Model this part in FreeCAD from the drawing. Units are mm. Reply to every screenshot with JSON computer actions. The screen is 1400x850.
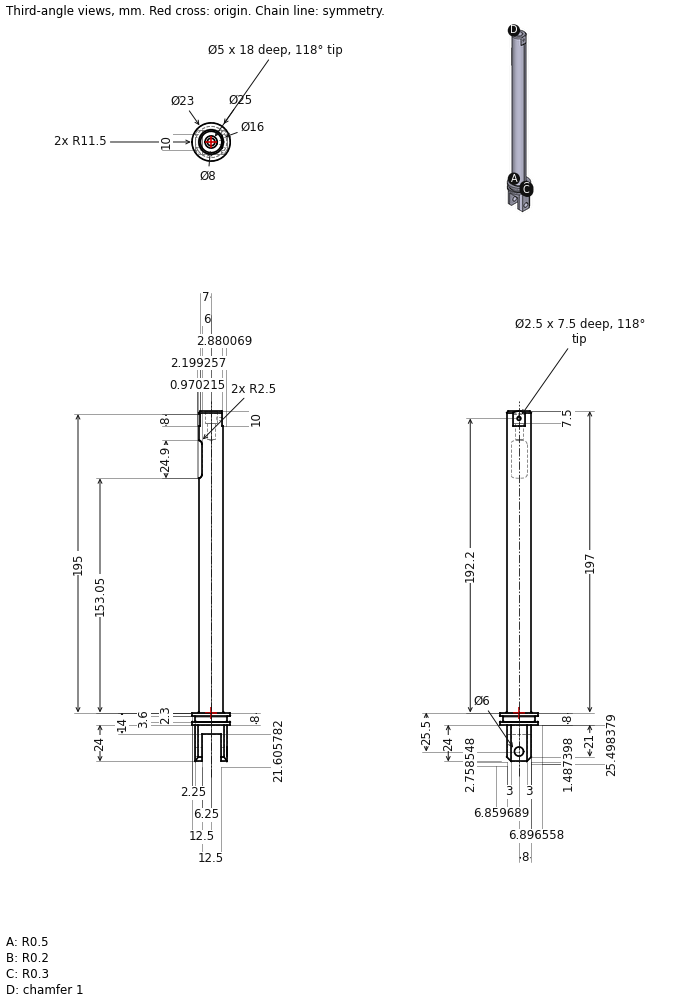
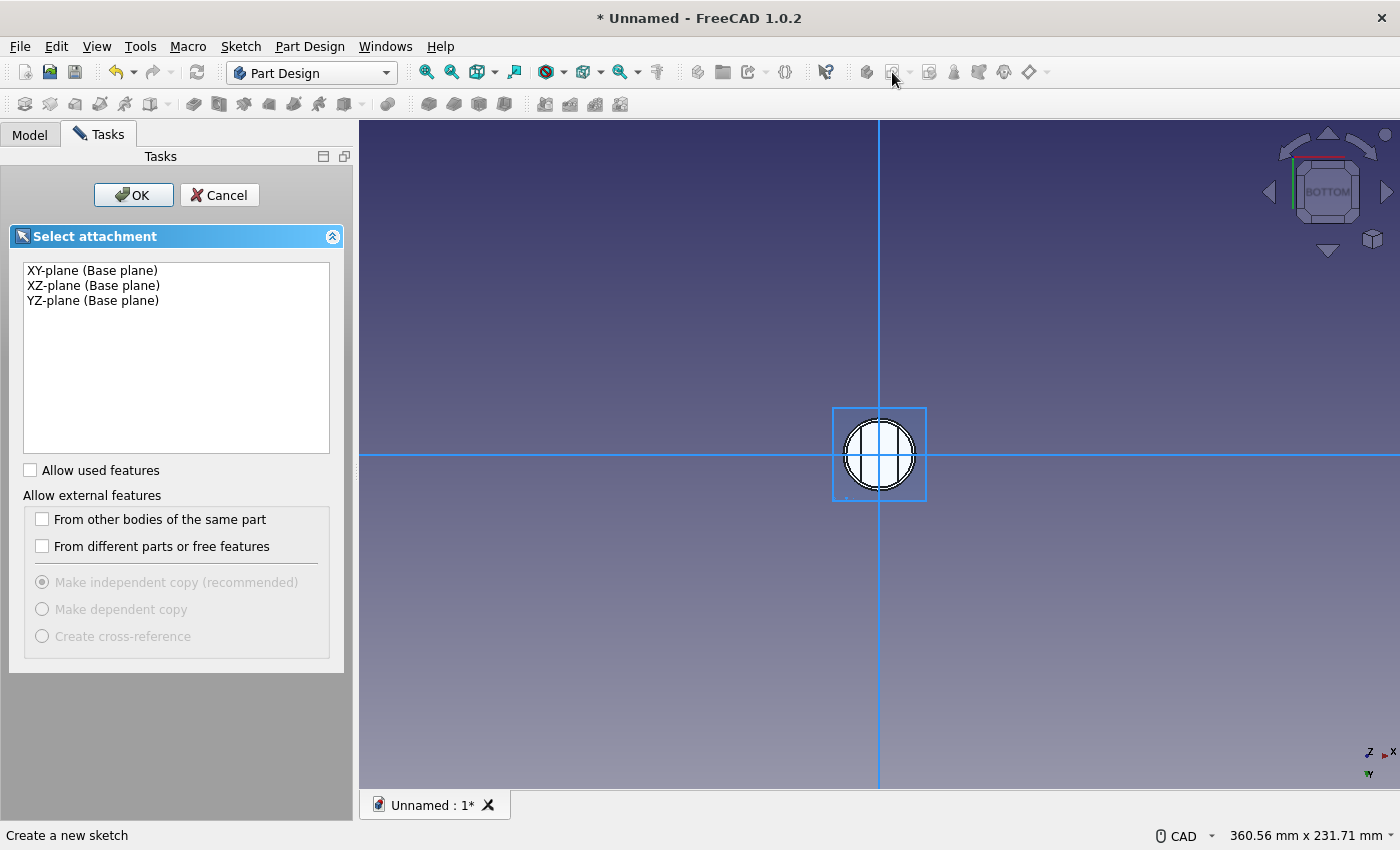
{"action": "left_click", "coordinate": [84, 300]}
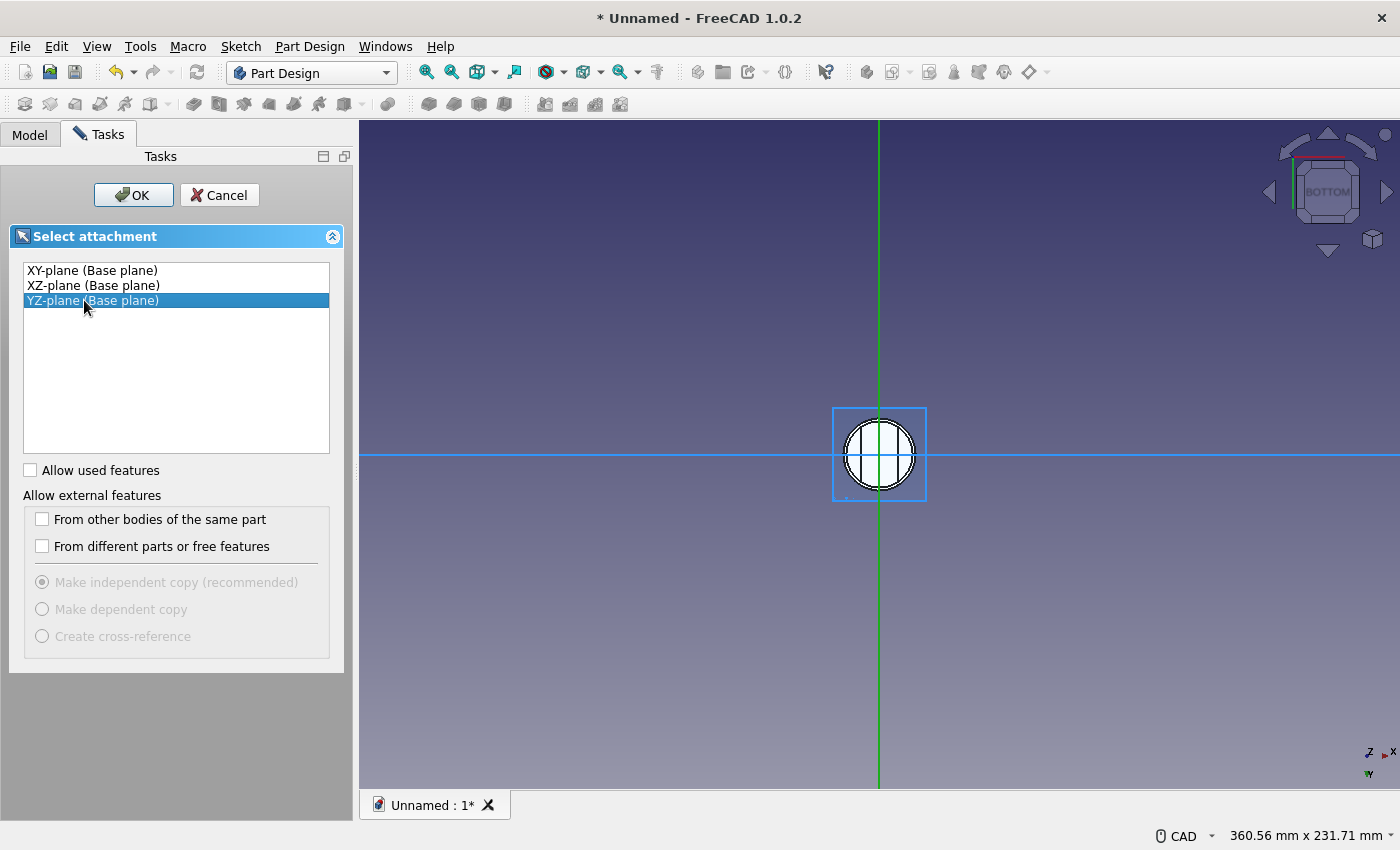
{"action": "left_click", "coordinate": [134, 195]}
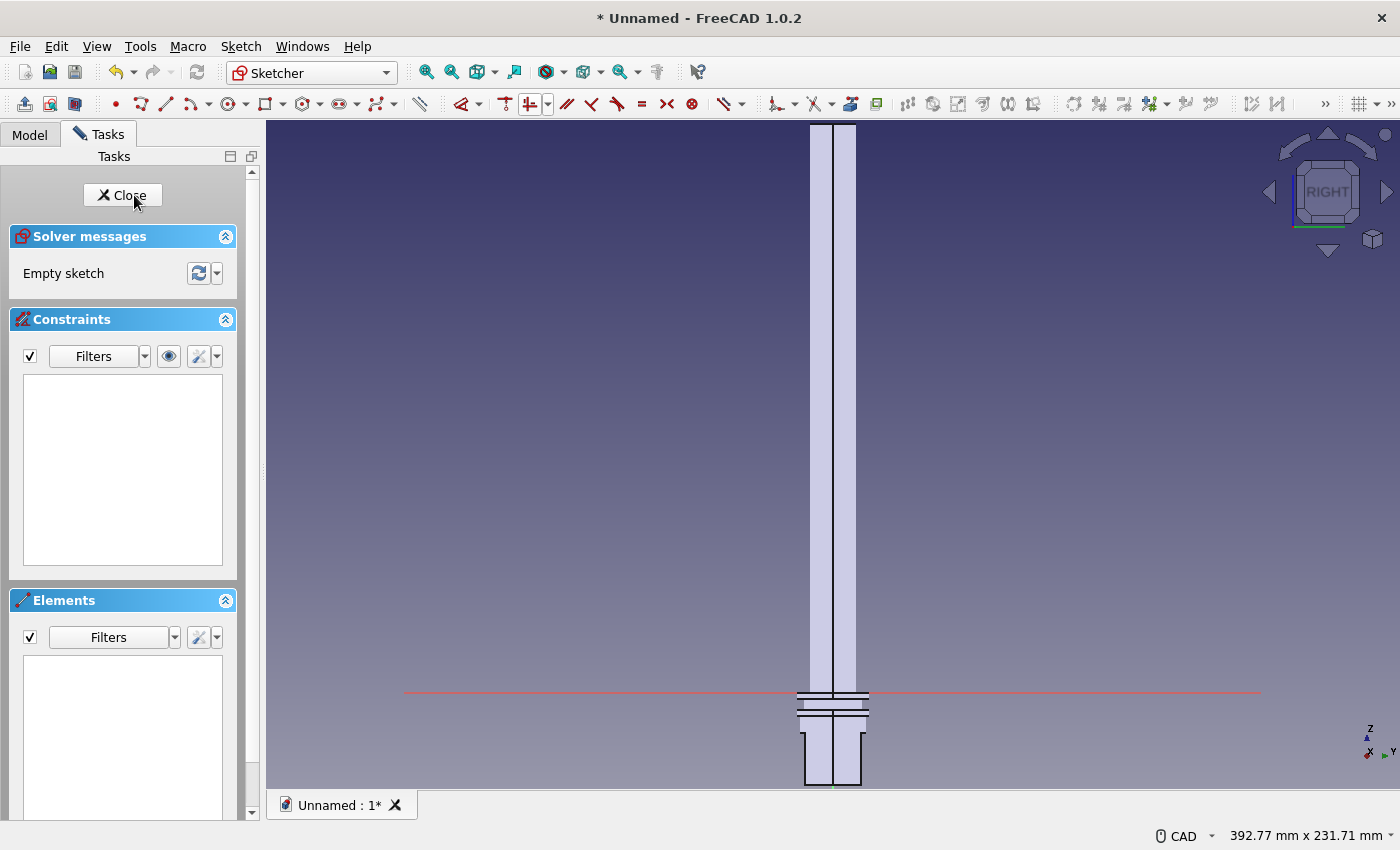
{"action": "left_click", "coordinate": [75, 104]}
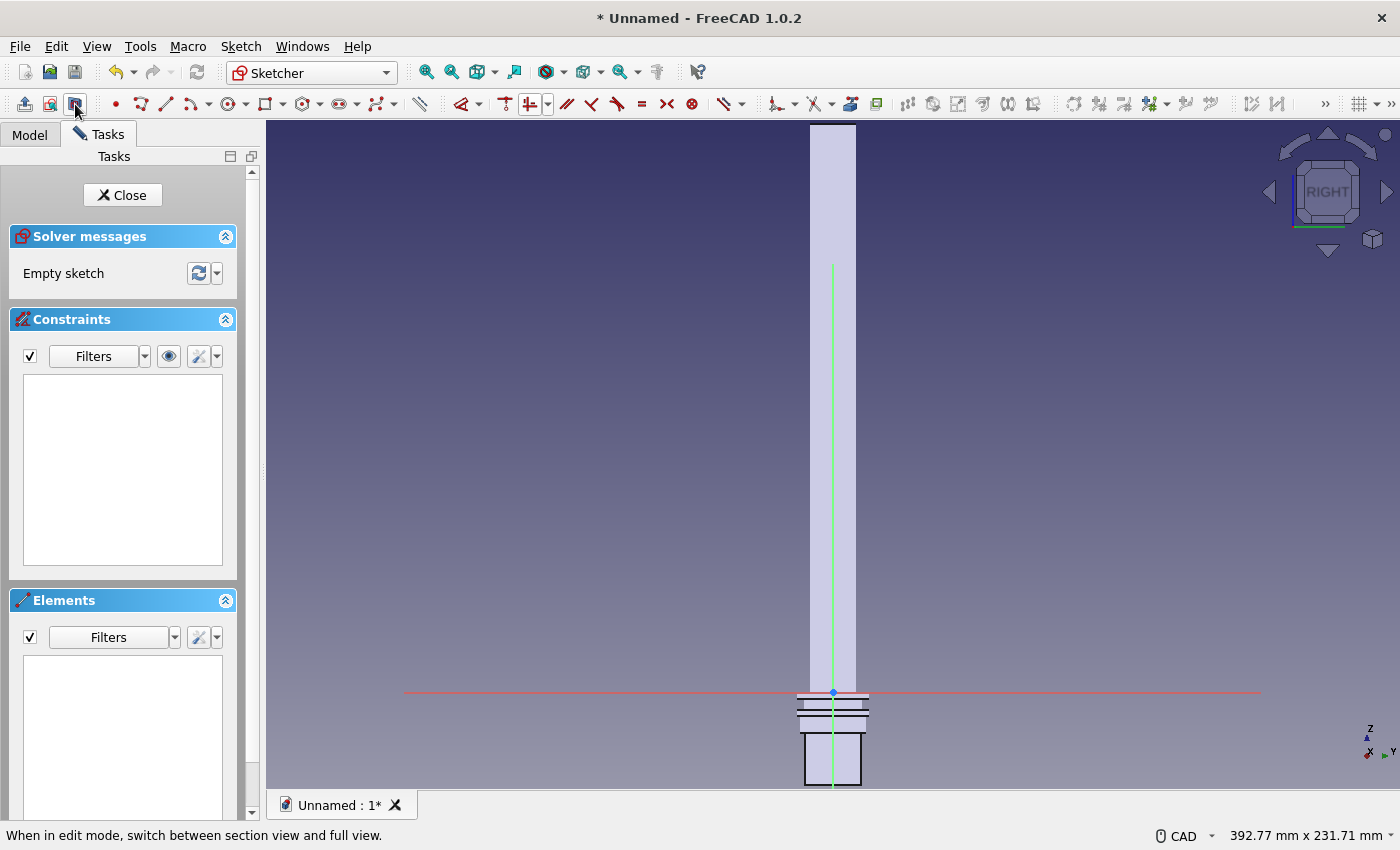
{"action": "scroll", "coordinate": [764, 454], "scroll_direction": "down", "scroll_amount": 5}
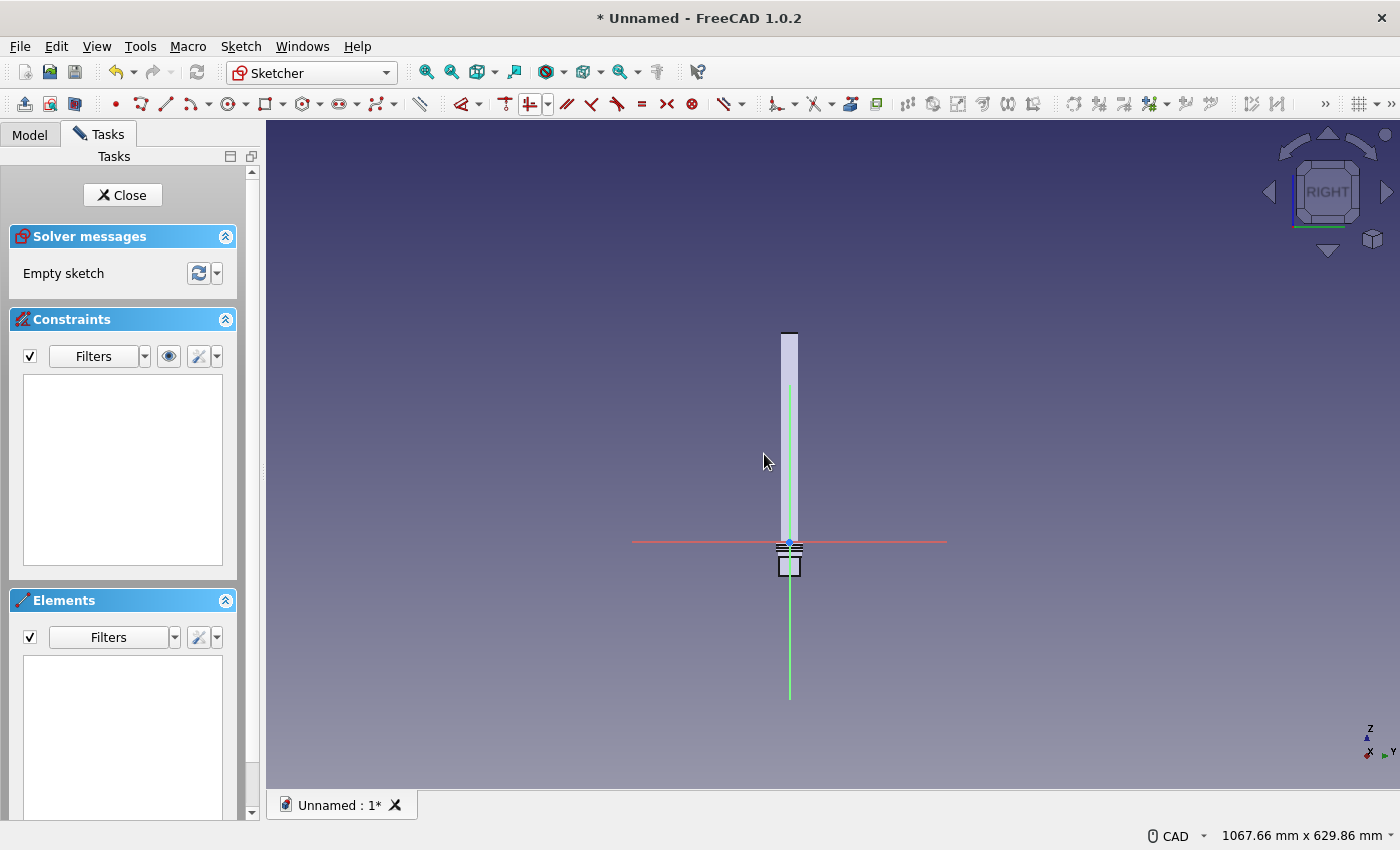
{"action": "scroll", "coordinate": [792, 571], "scroll_direction": "up", "scroll_amount": 12}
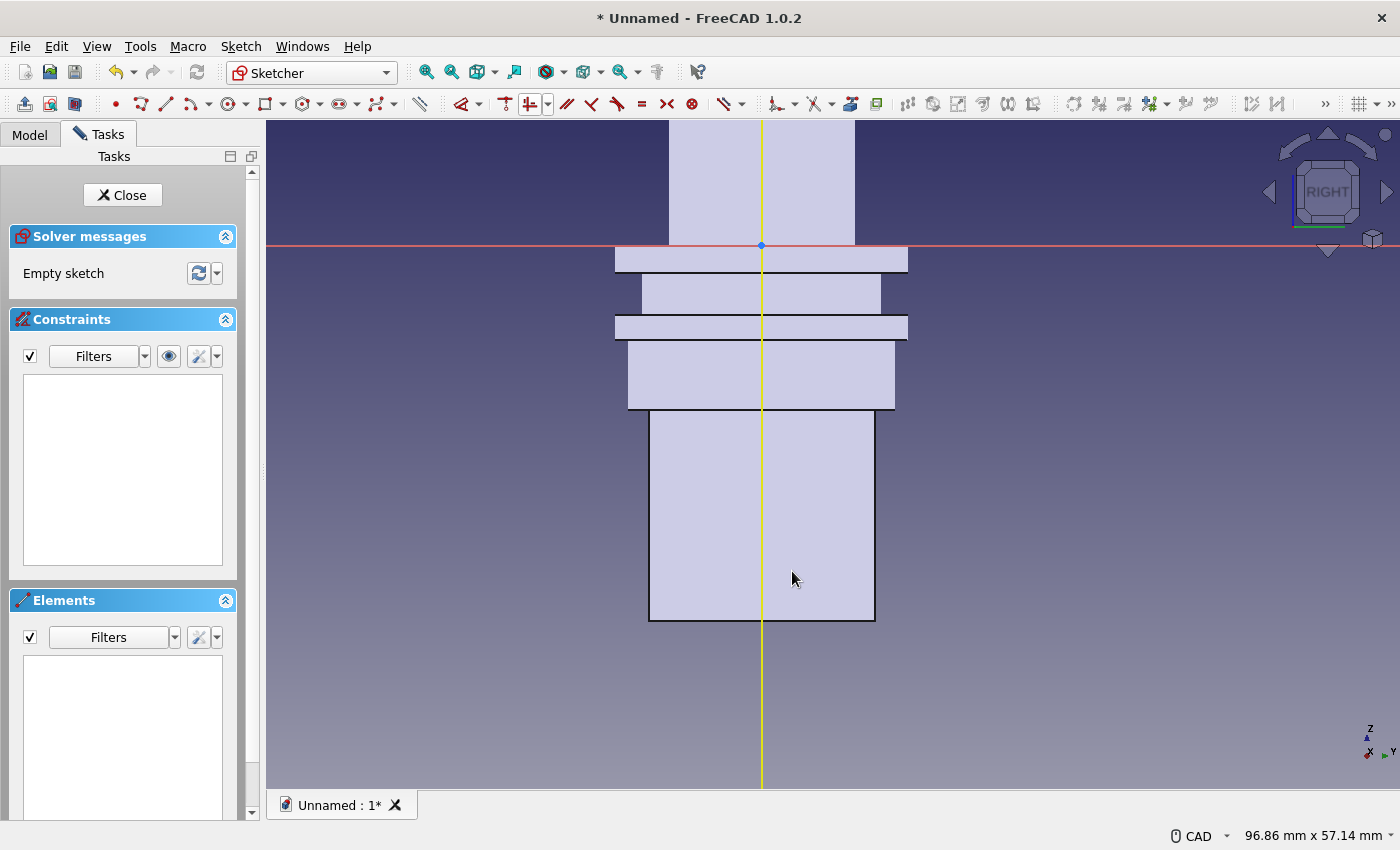
{"action": "left_click", "coordinate": [141, 104]}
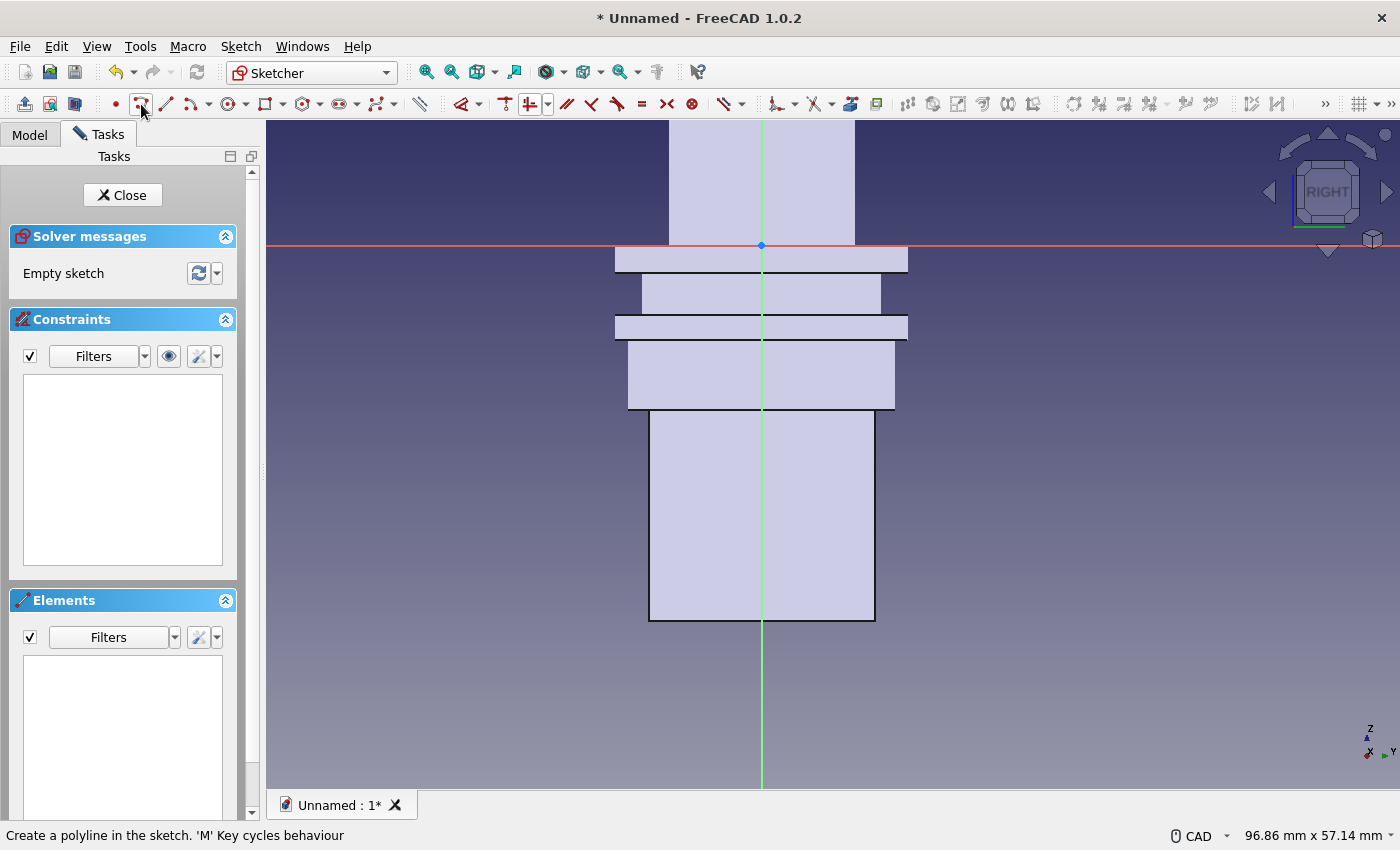
{"action": "left_click", "coordinate": [855, 340]}
{"action": "left_click", "coordinate": [936, 340]}
{"action": "left_click", "coordinate": [936, 638]}
{"action": "left_click", "coordinate": [855, 638]}
{"action": "left_click", "coordinate": [855, 621]}
{"action": "left_click", "coordinate": [820, 621]}
{"action": "left_click", "coordinate": [855, 585]}
{"action": "left_click", "coordinate": [855, 341]}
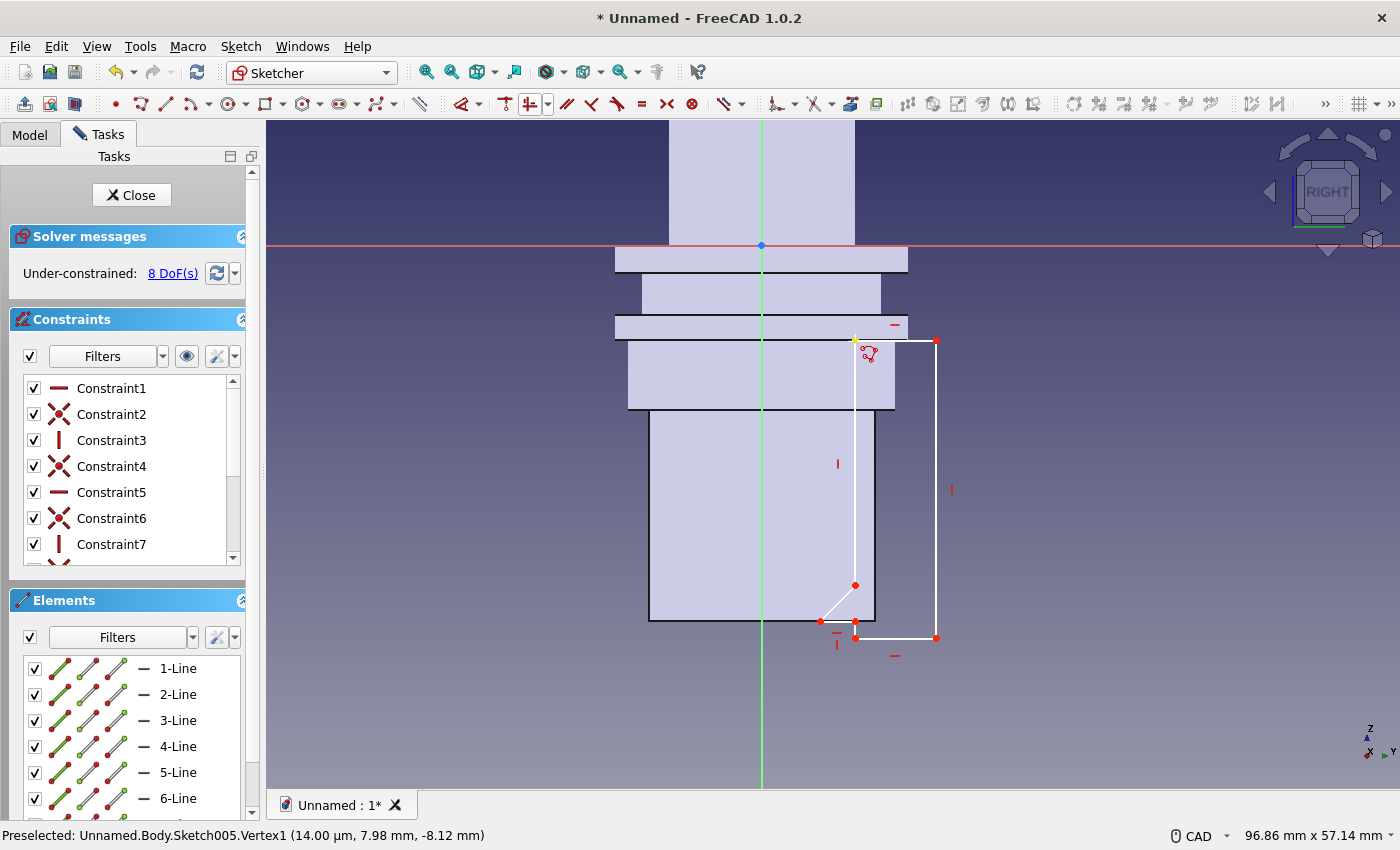
{"action": "left_click", "coordinate": [668, 340]}
{"action": "left_click", "coordinate": [668, 585]}
{"action": "left_click", "coordinate": [703, 621]}
{"action": "left_click", "coordinate": [668, 621]}
{"action": "left_click", "coordinate": [668, 653]}
{"action": "left_click", "coordinate": [588, 653]}
{"action": "left_click", "coordinate": [588, 340]}
{"action": "left_click", "coordinate": [668, 341]}
{"action": "key", "text": "Escape"}
{"action": "key", "text": "Escape"}